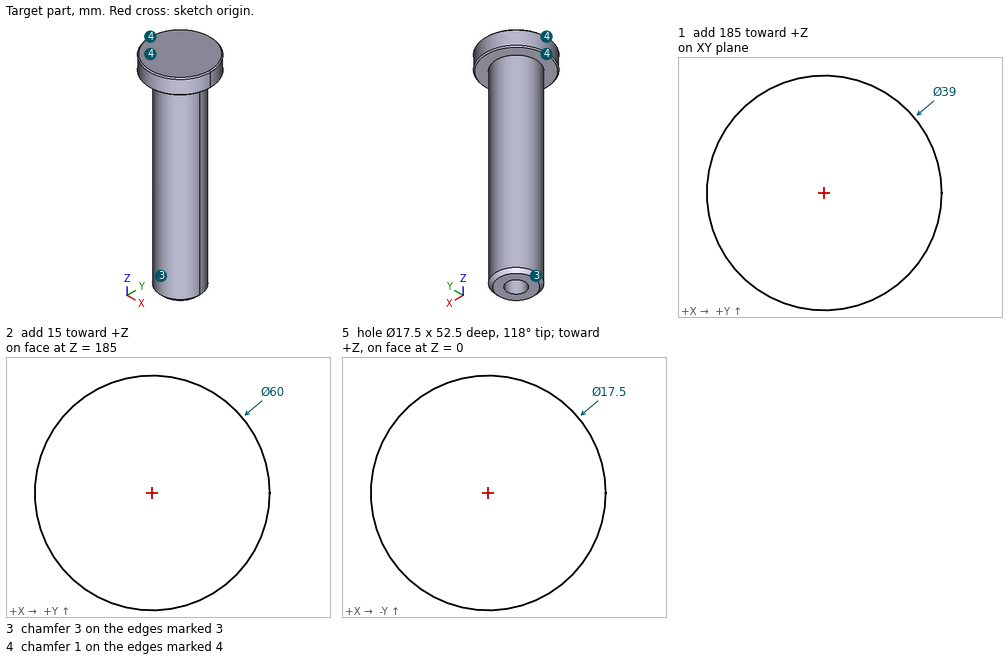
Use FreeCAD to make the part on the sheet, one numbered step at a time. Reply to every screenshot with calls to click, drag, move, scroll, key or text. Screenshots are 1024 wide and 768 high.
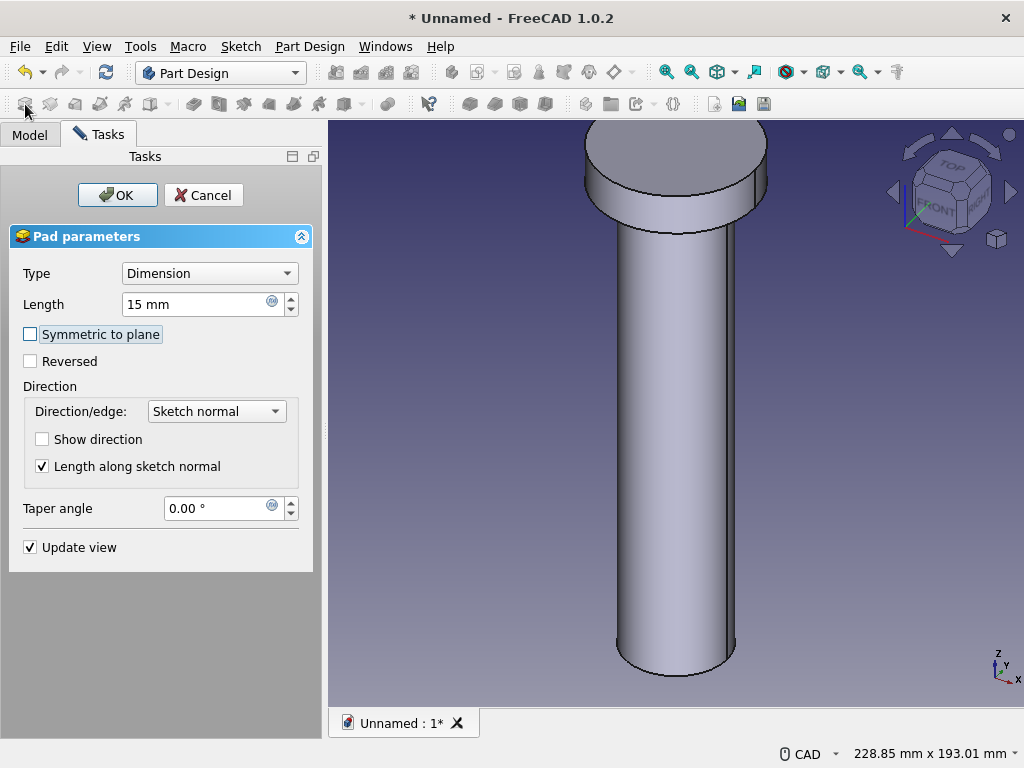
click(118, 195)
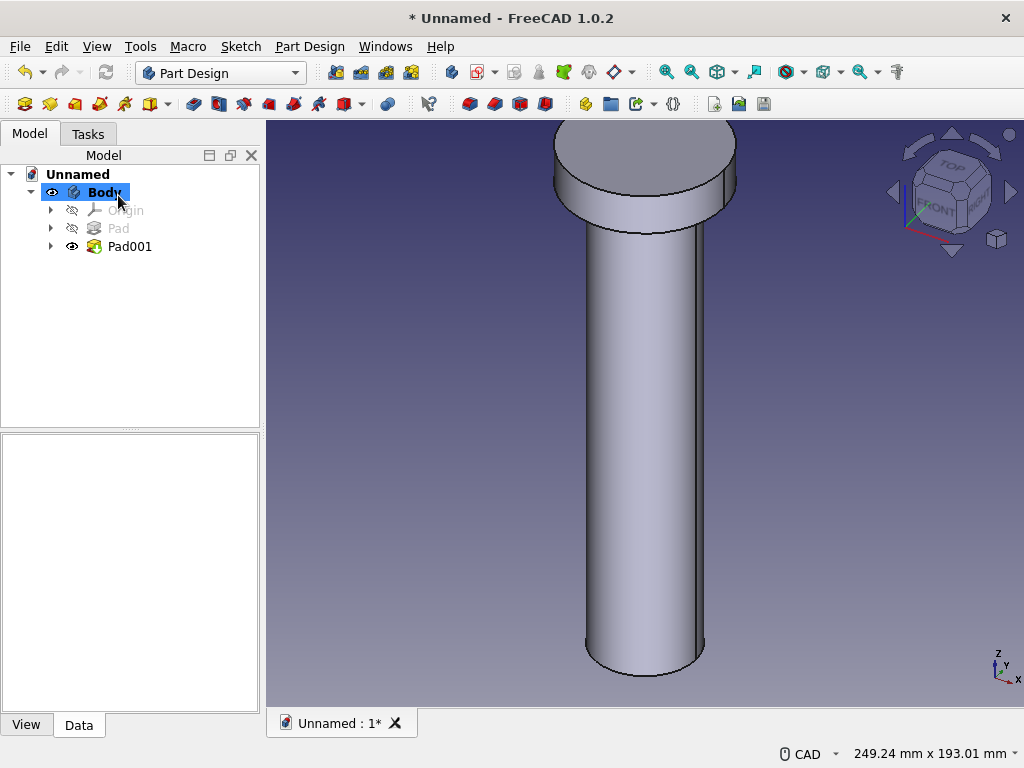
key(v)
key(f)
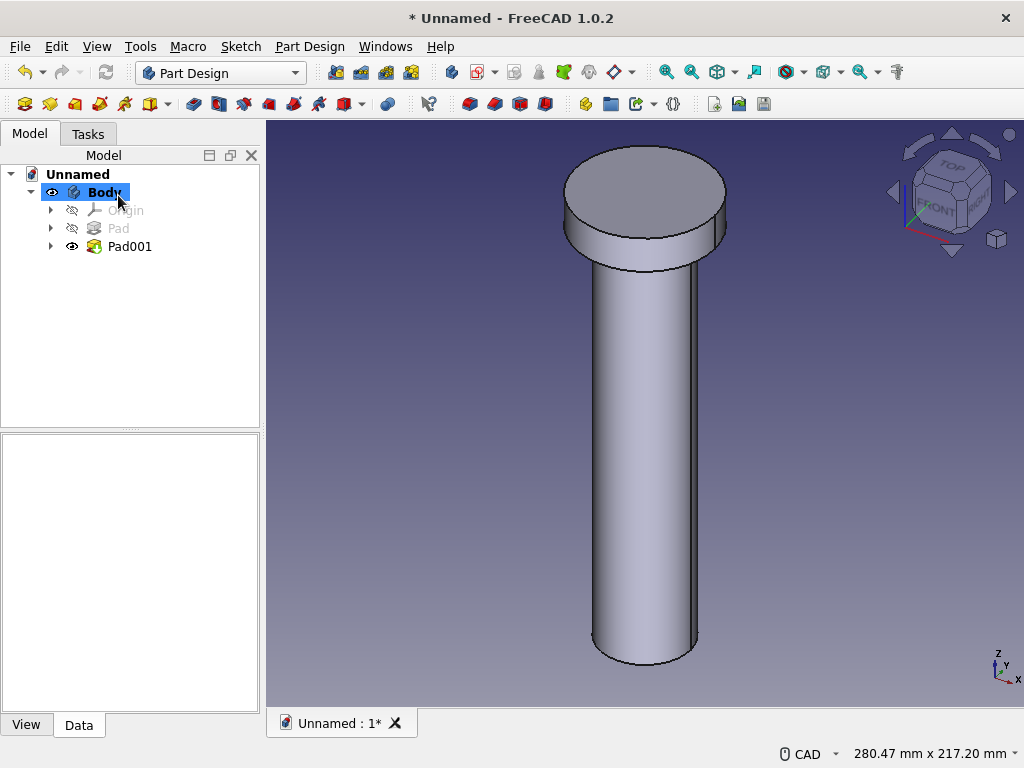
key(0)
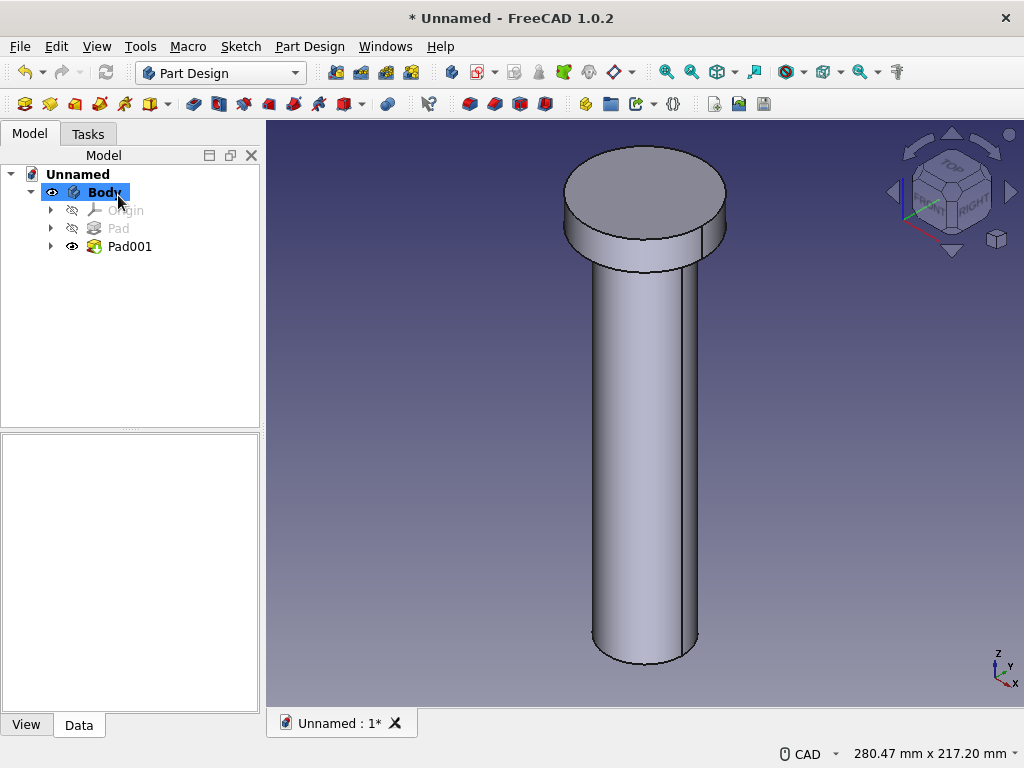
key(2)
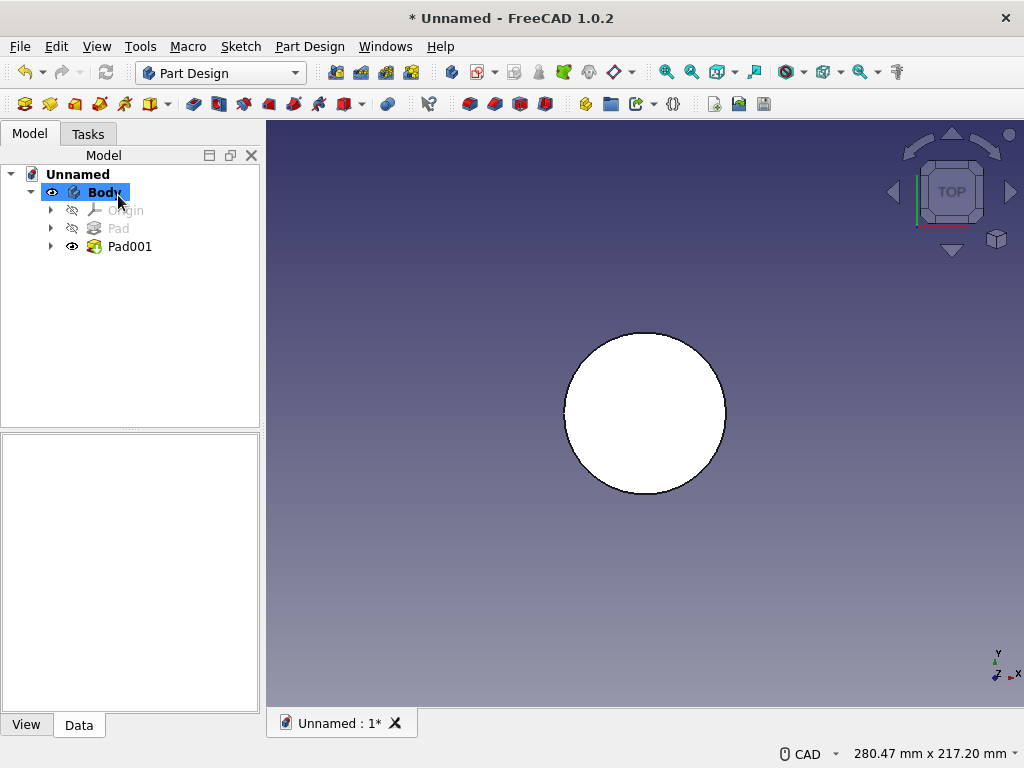
click(667, 72)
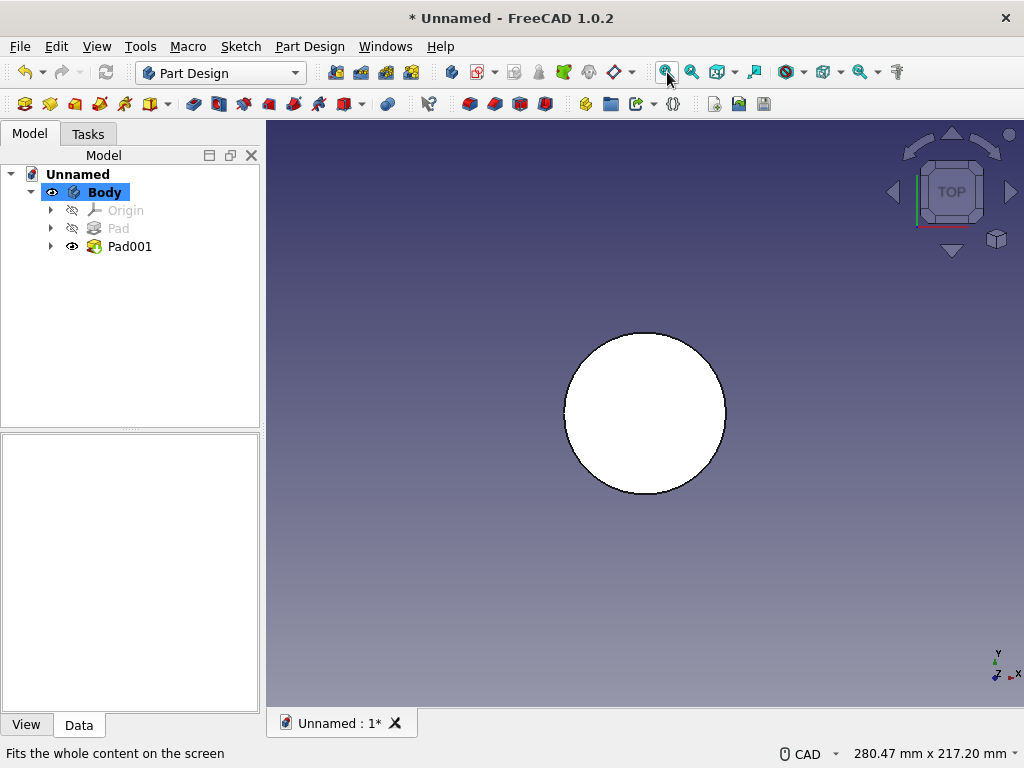
key(1)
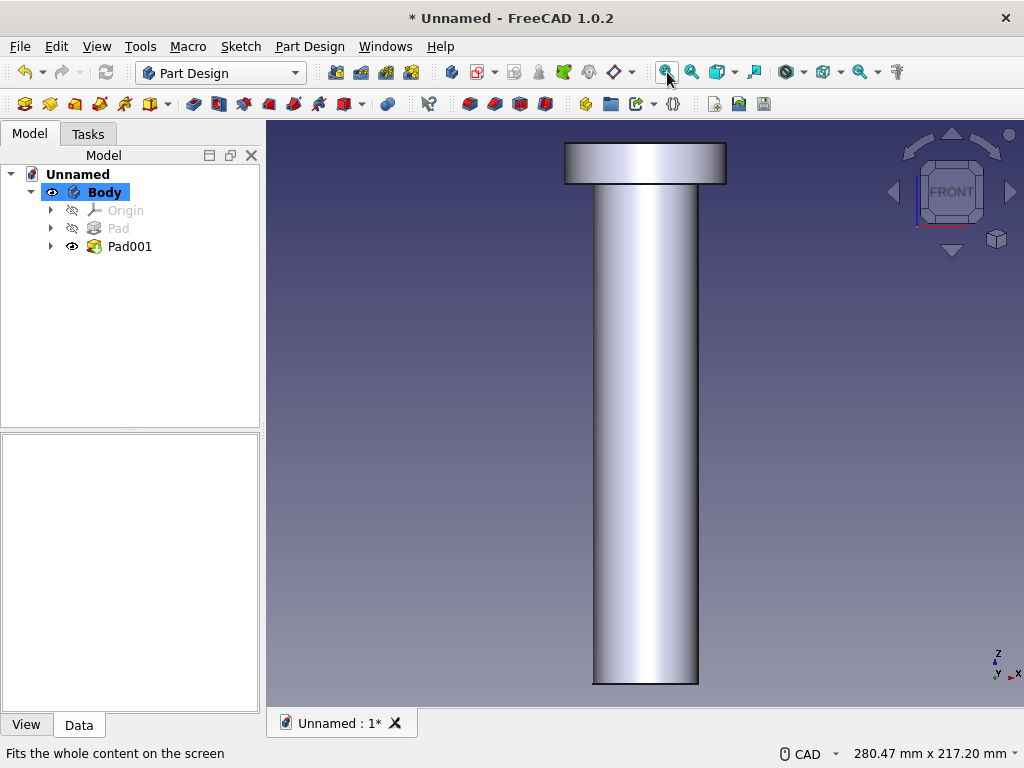
key(3)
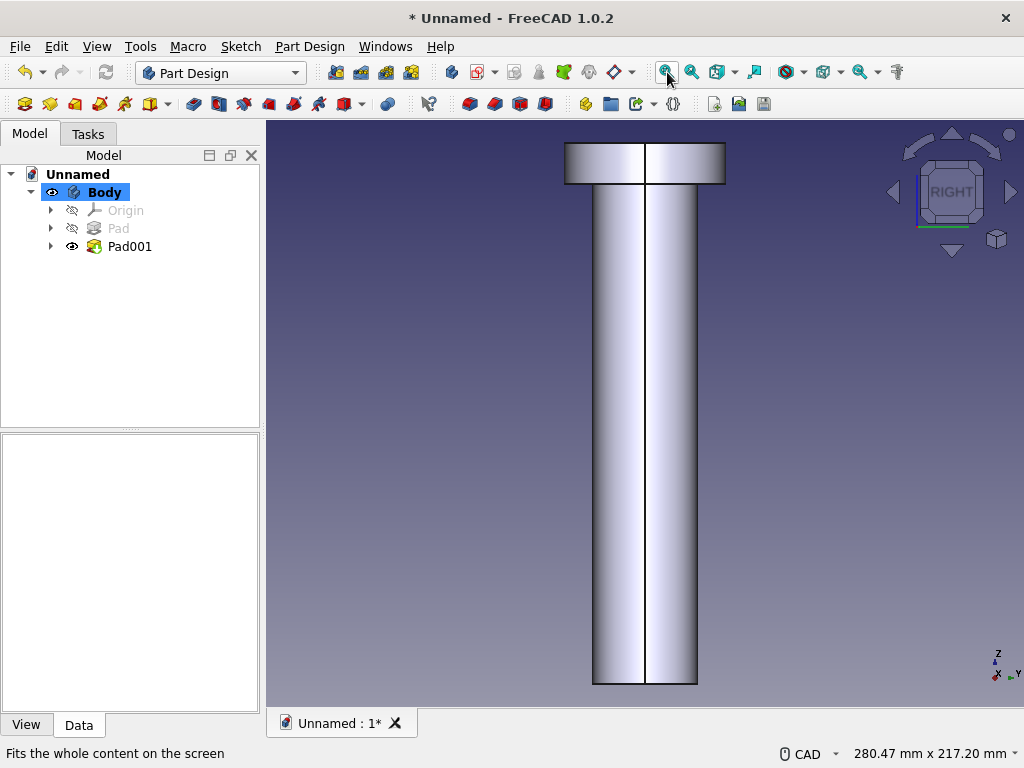
key(5)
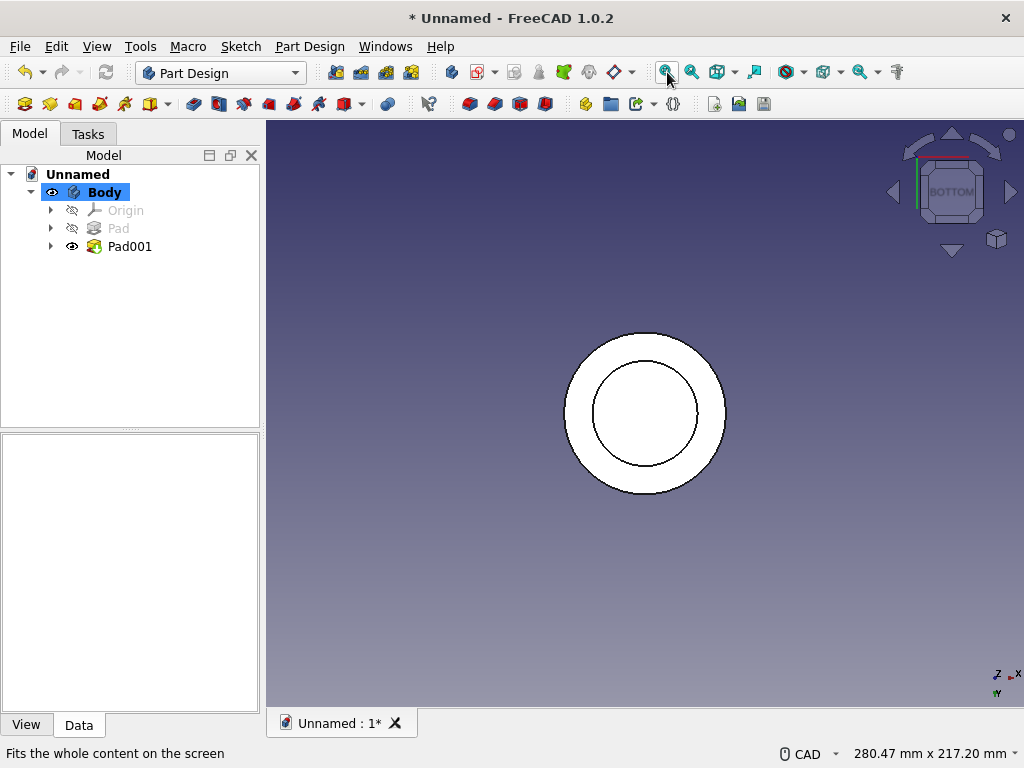
key(v)
key(f)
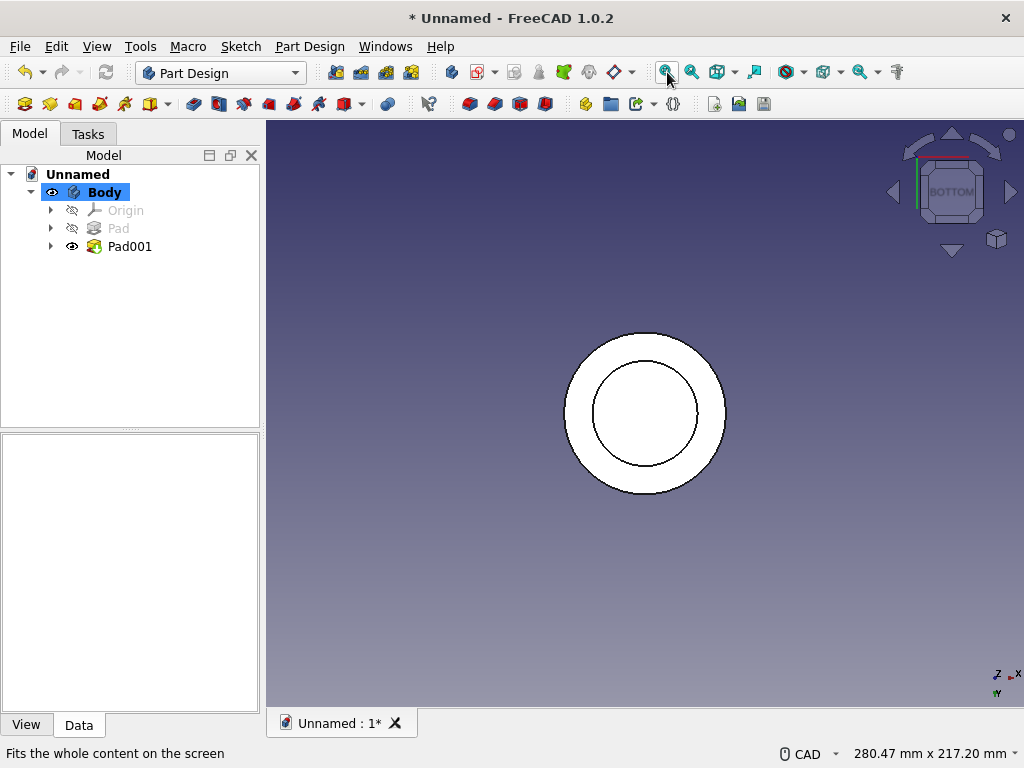
click(602, 443)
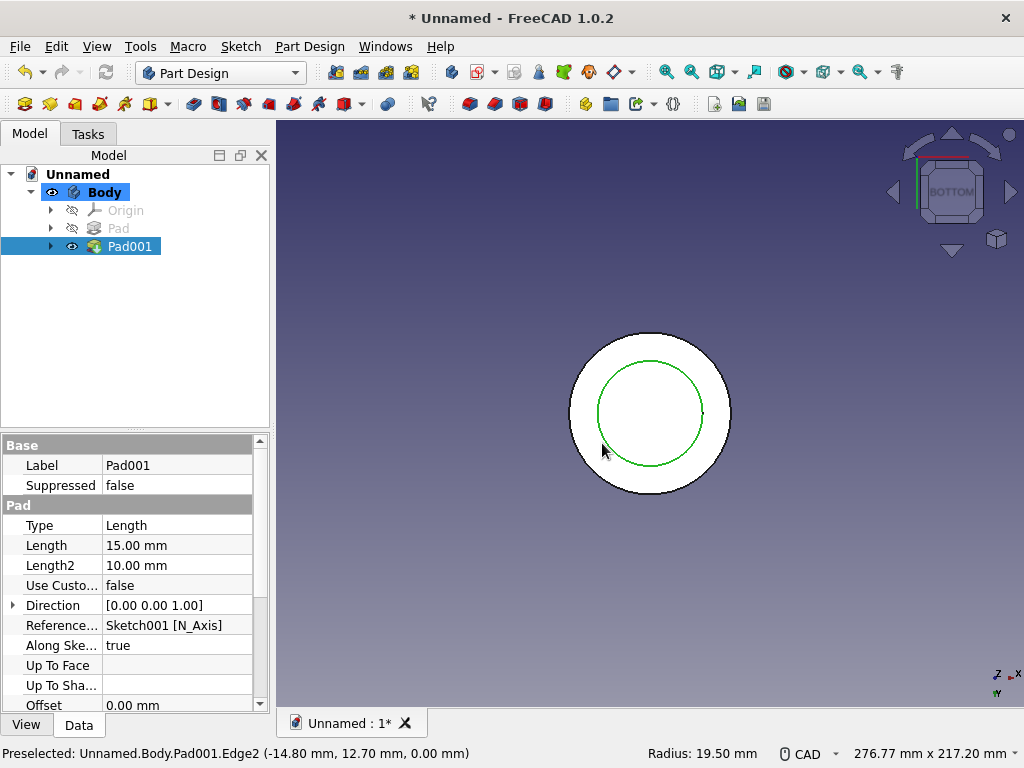
click(495, 104)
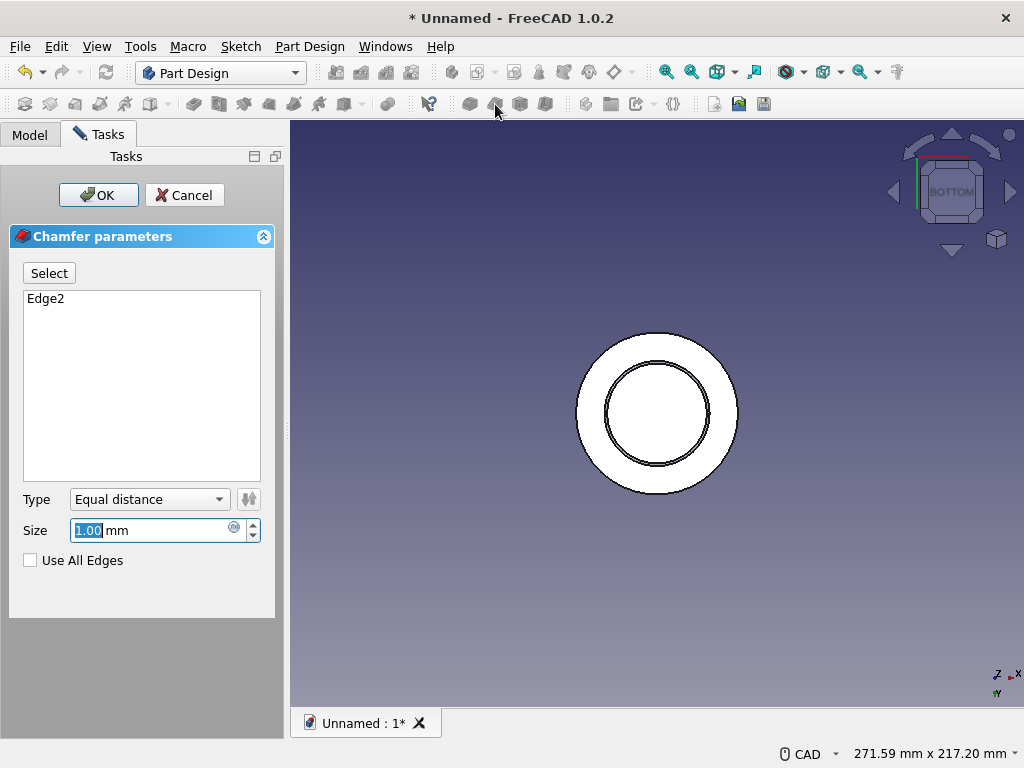
text(3)
key(Tab)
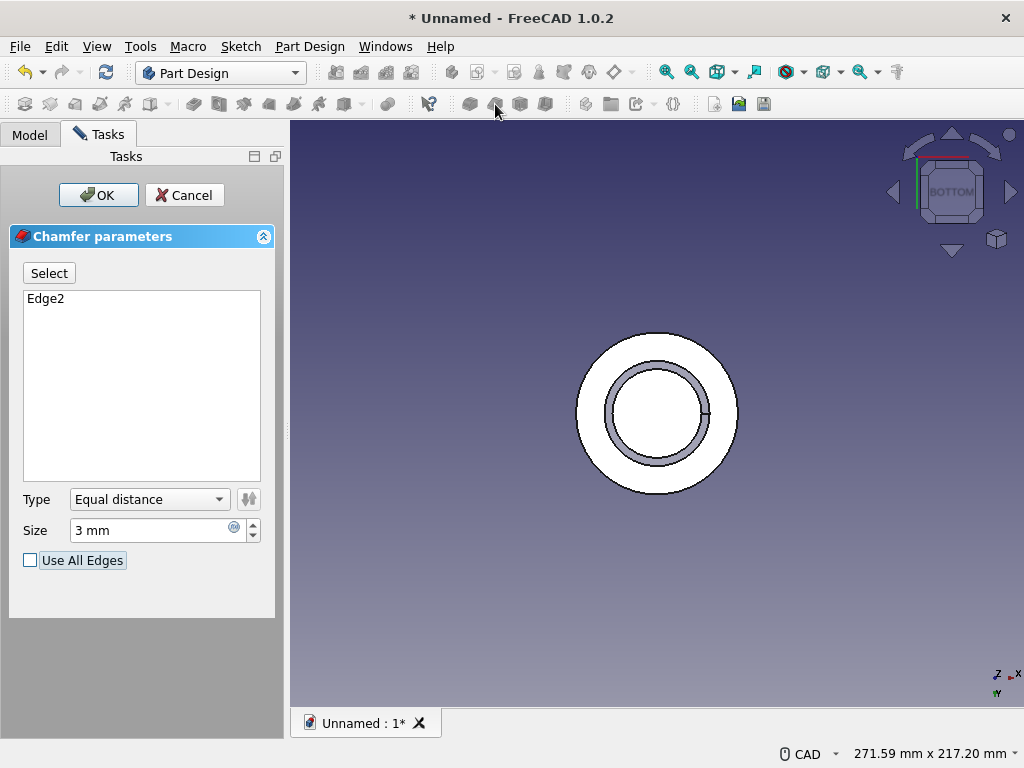
click(99, 195)